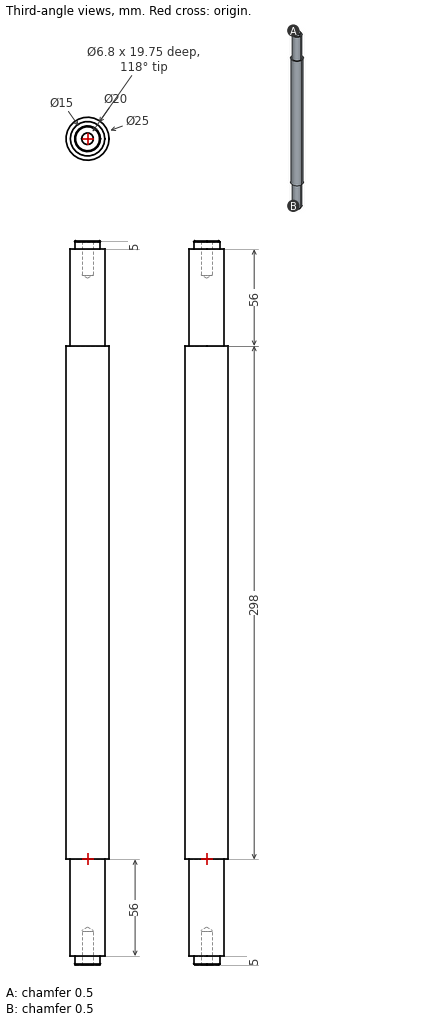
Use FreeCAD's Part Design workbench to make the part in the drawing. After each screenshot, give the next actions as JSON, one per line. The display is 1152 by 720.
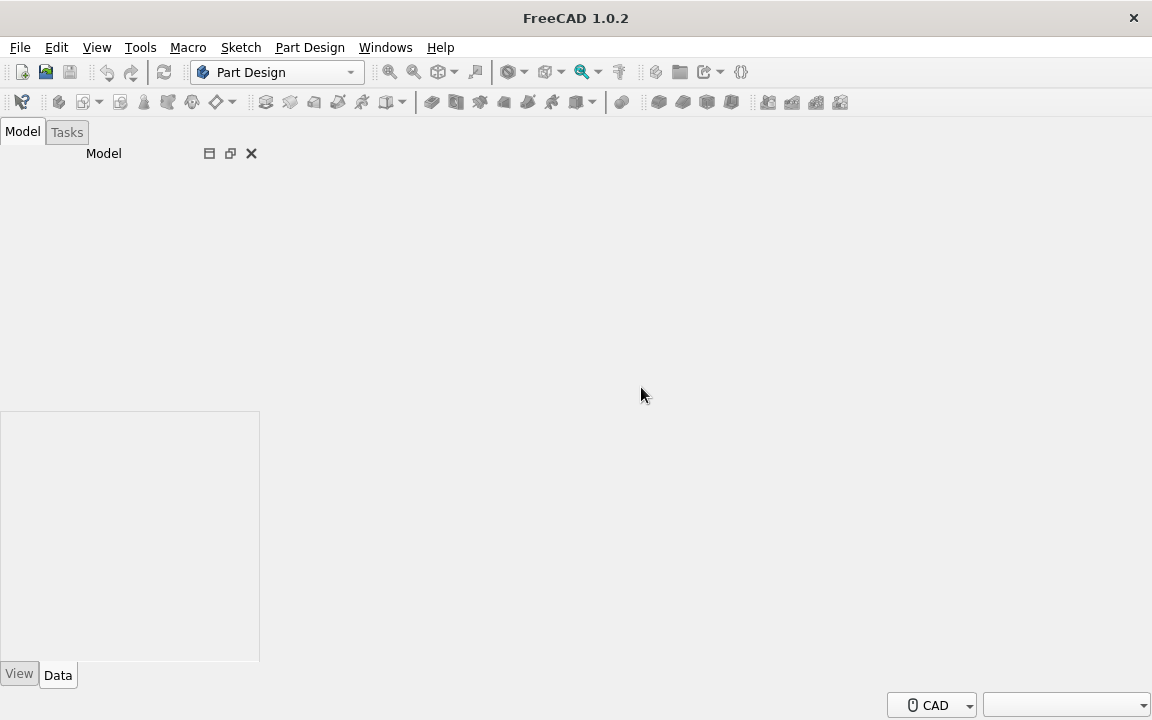
{"action": "left_click", "coordinate": [22, 72]}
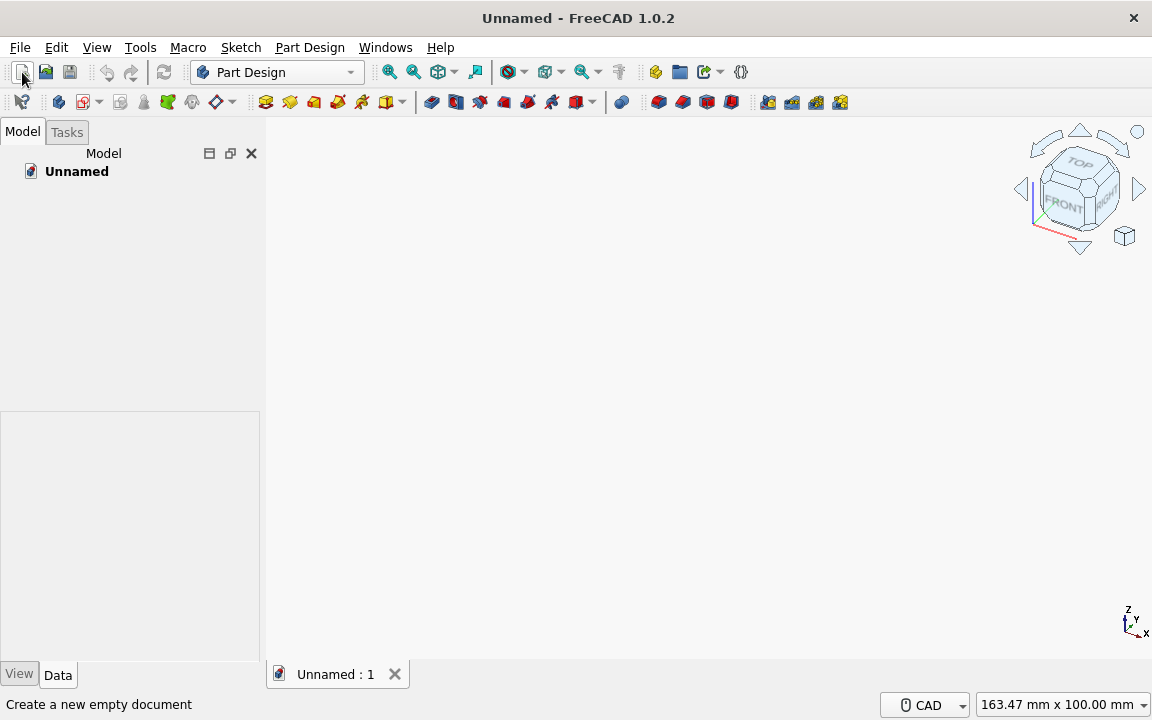
{"action": "left_click", "coordinate": [84, 102]}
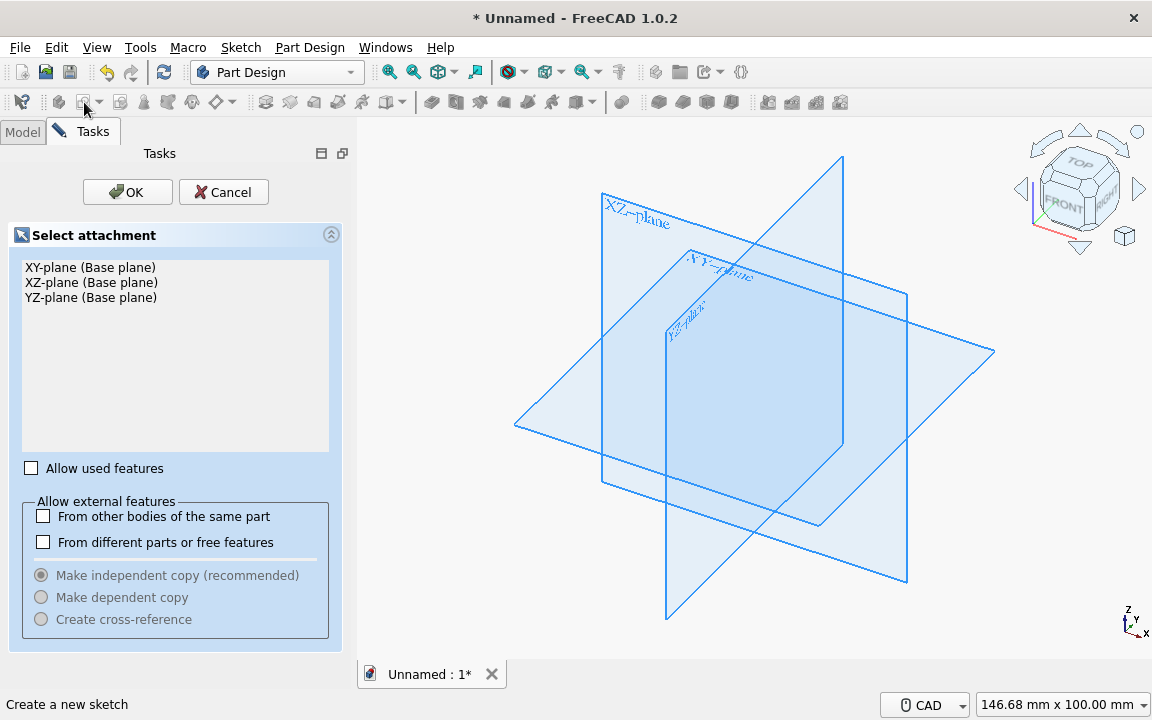
{"action": "left_click", "coordinate": [82, 268]}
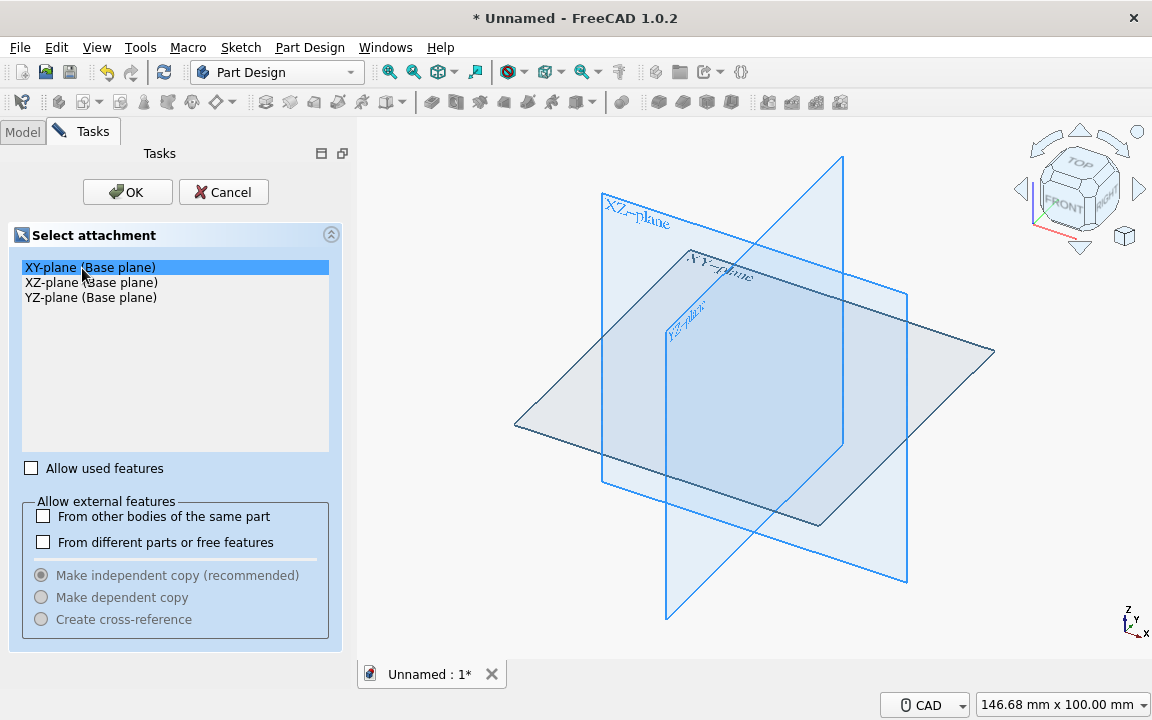
{"action": "left_click", "coordinate": [128, 192]}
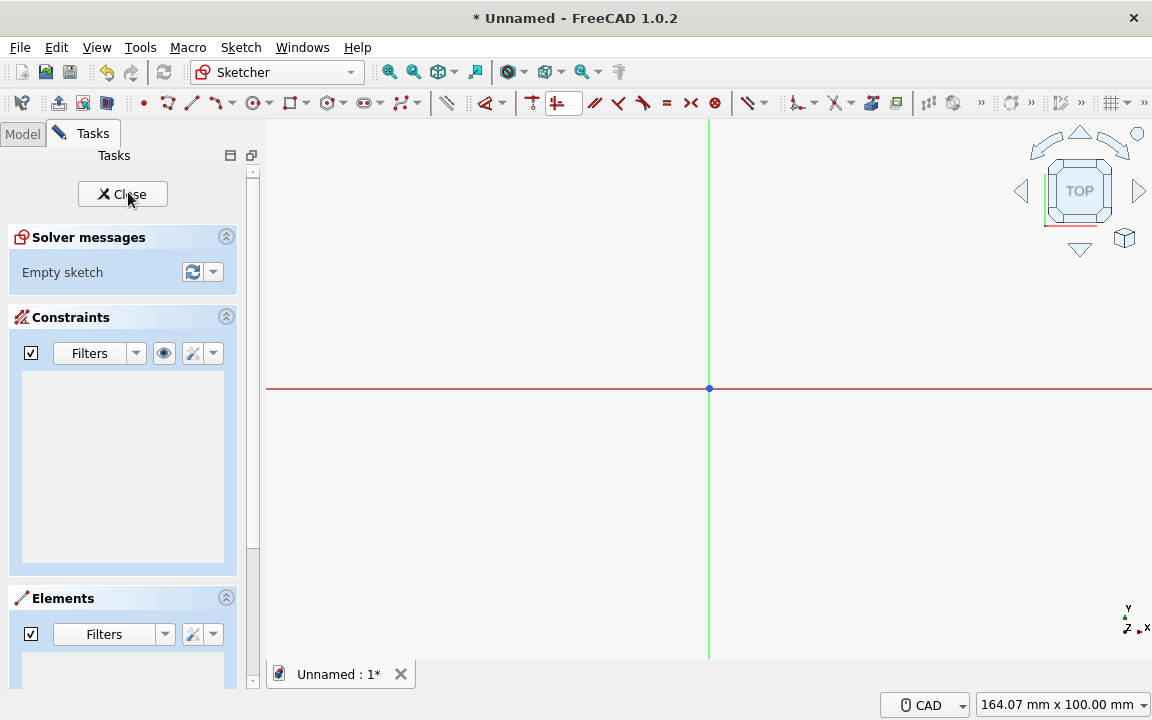
{"action": "scroll", "coordinate": [749, 389], "scroll_direction": "up", "scroll_amount": 5}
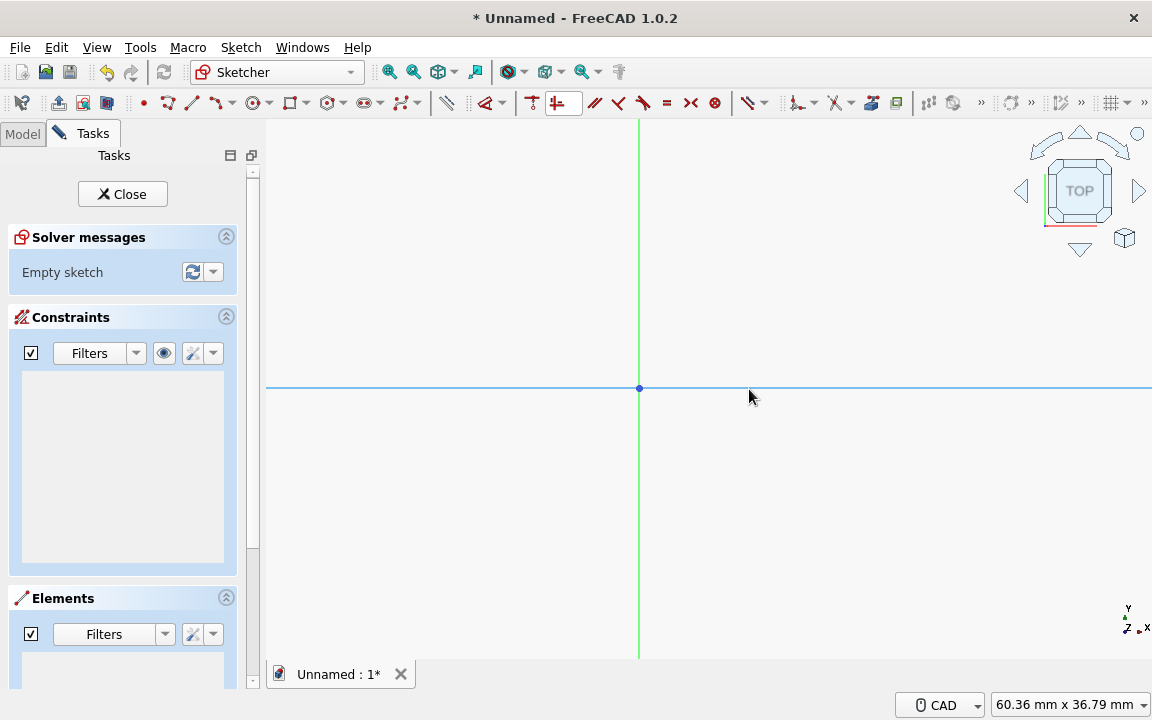
{"action": "left_click", "coordinate": [254, 104]}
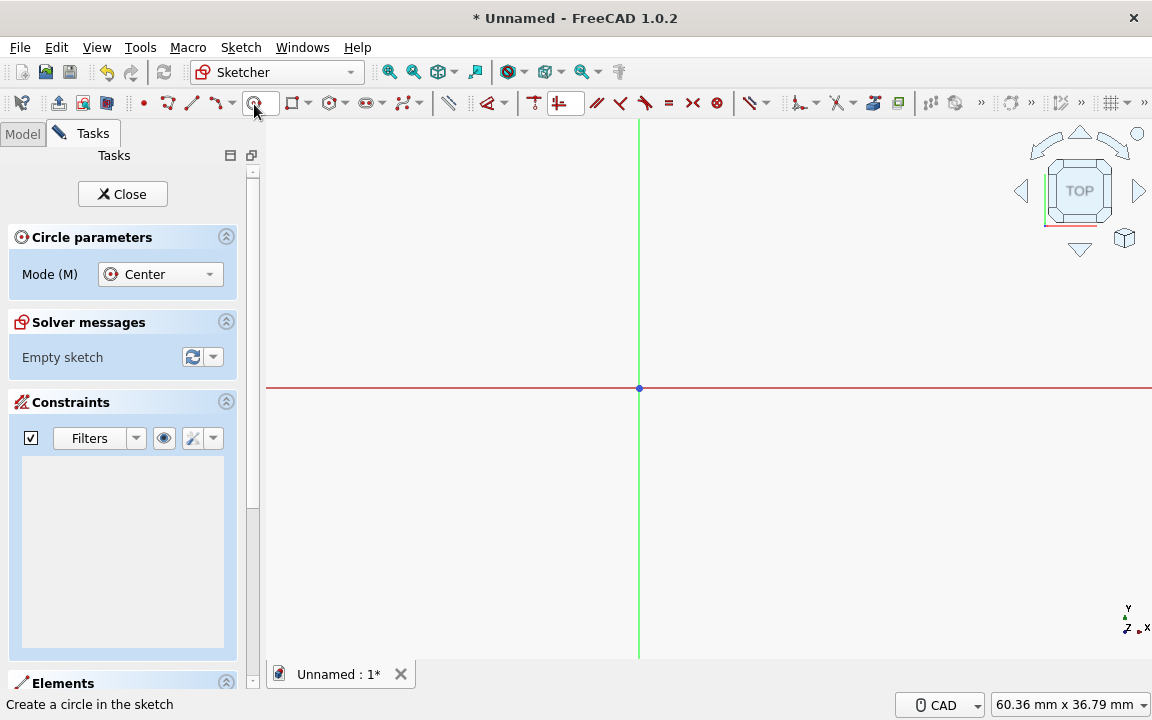
{"action": "left_click", "coordinate": [639, 388]}
{"action": "left_click", "coordinate": [769, 258]}
{"action": "key", "text": "Escape"}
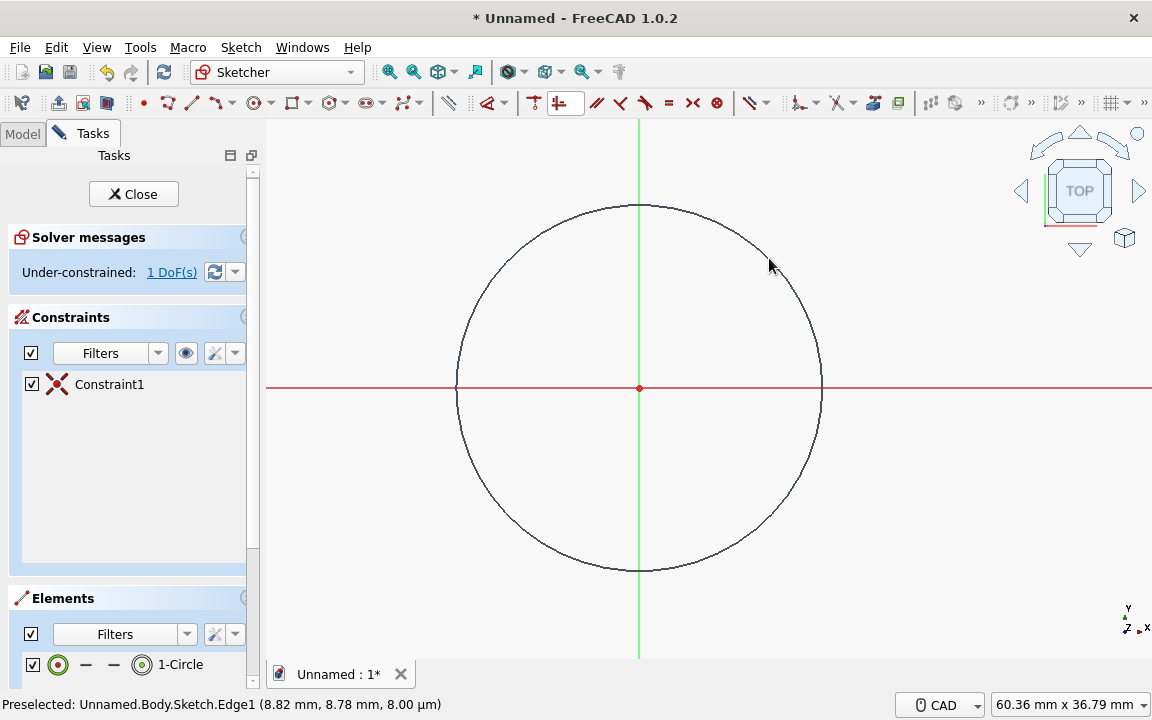
{"action": "left_click", "coordinate": [488, 104]}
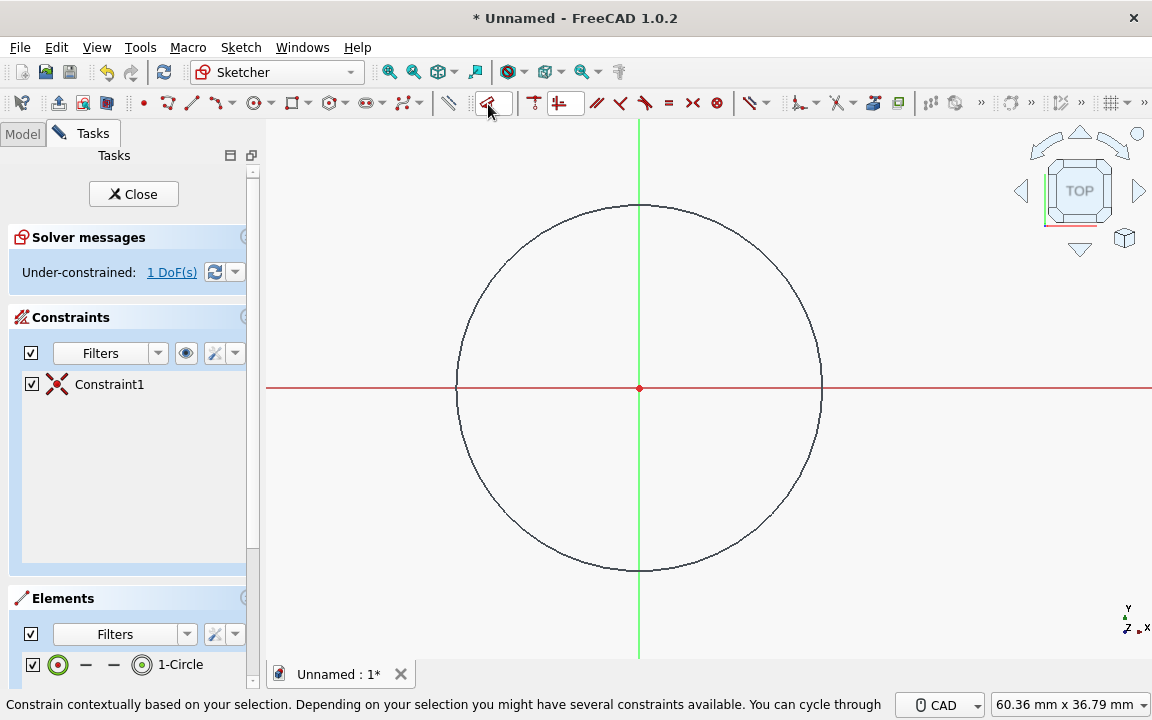
{"action": "left_click", "coordinate": [768, 258]}
{"action": "left_click", "coordinate": [790, 235]}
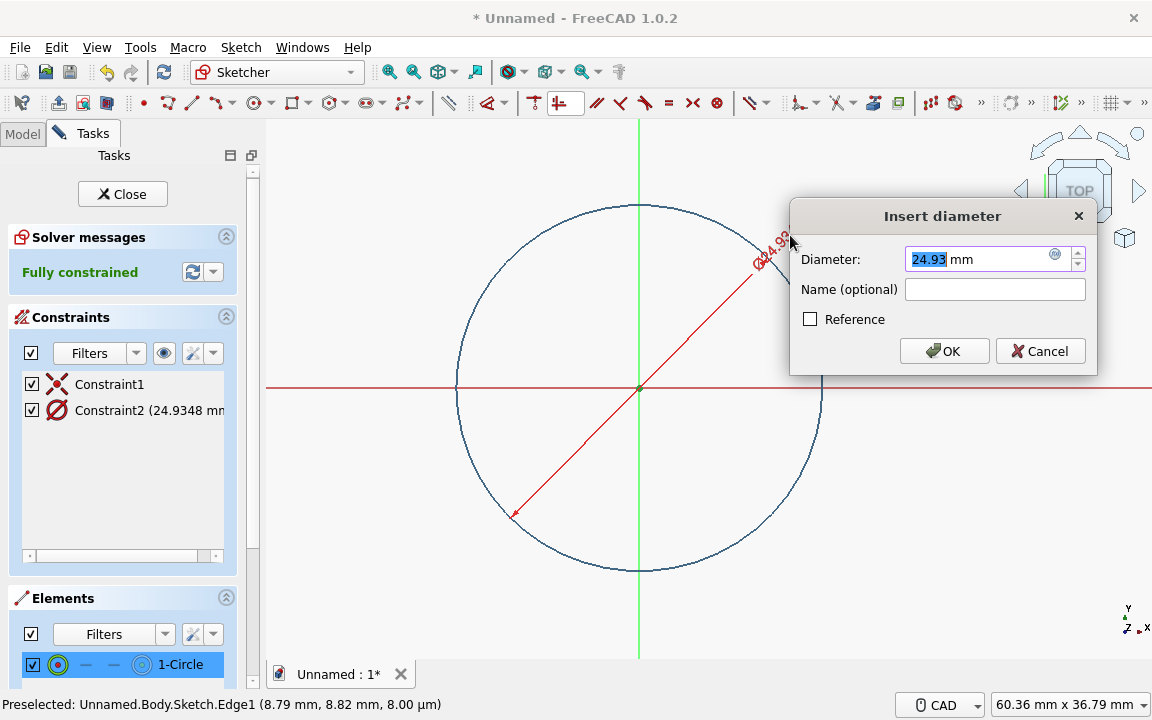
{"action": "type", "text": "25"}
{"action": "key", "text": "Return"}
{"action": "key", "text": "Escape"}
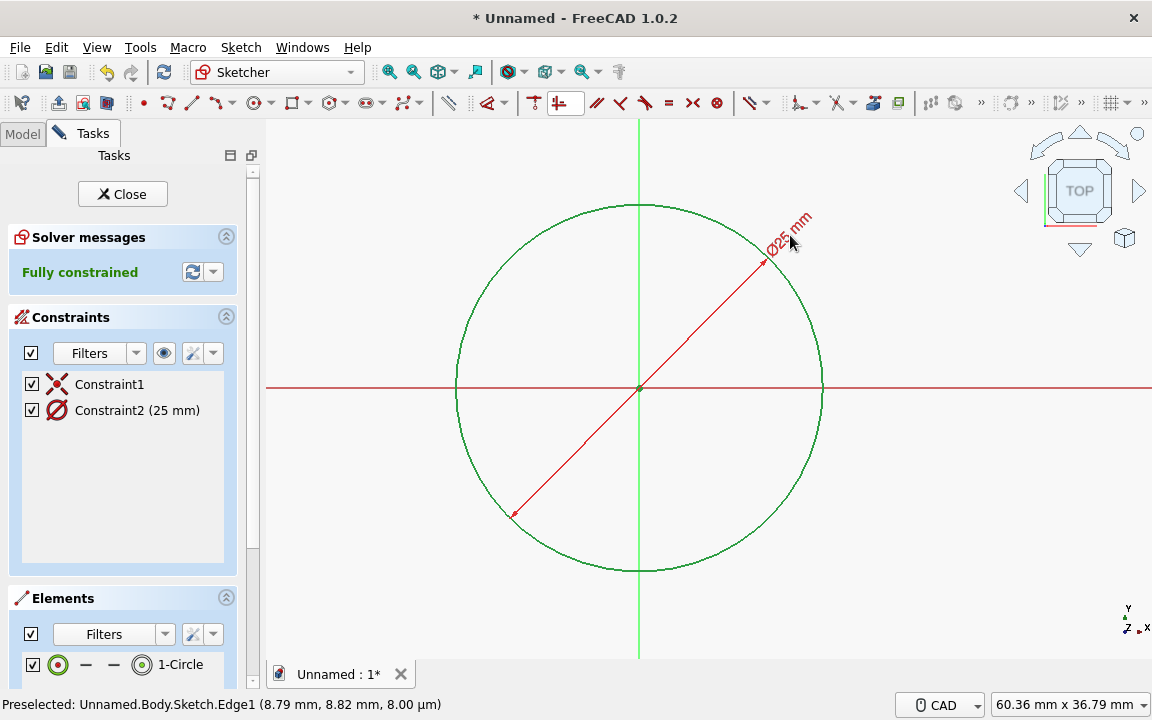
{"action": "left_click", "coordinate": [123, 194]}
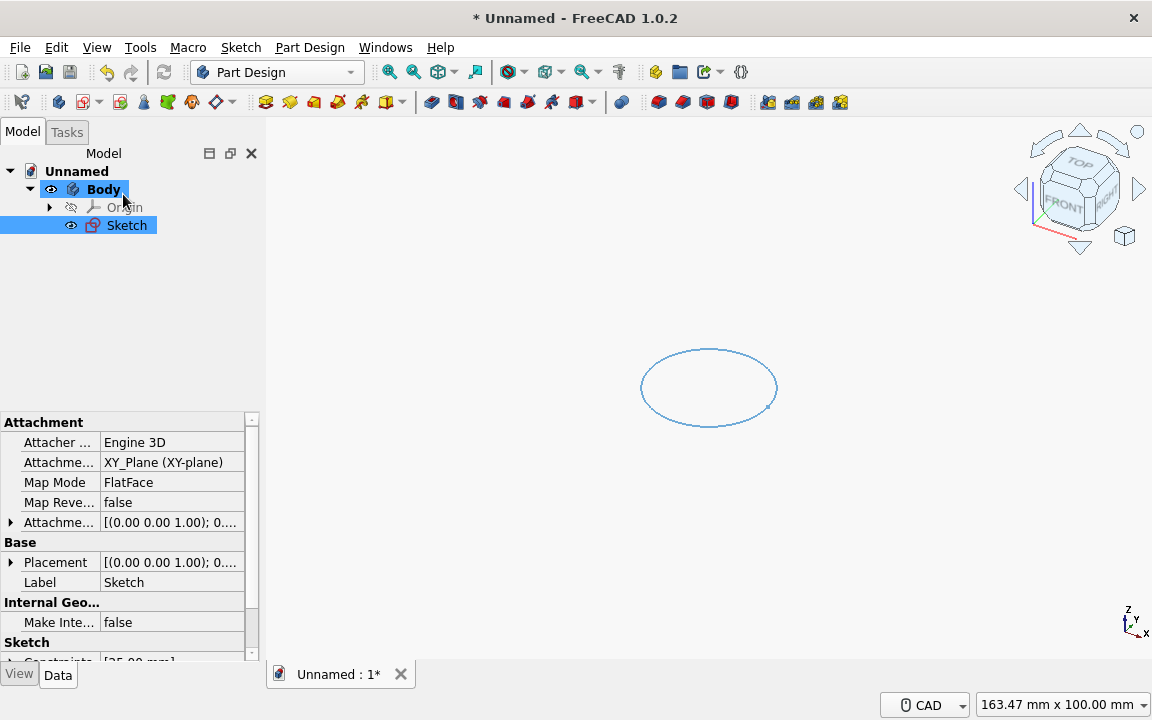
{"action": "left_click", "coordinate": [266, 102]}